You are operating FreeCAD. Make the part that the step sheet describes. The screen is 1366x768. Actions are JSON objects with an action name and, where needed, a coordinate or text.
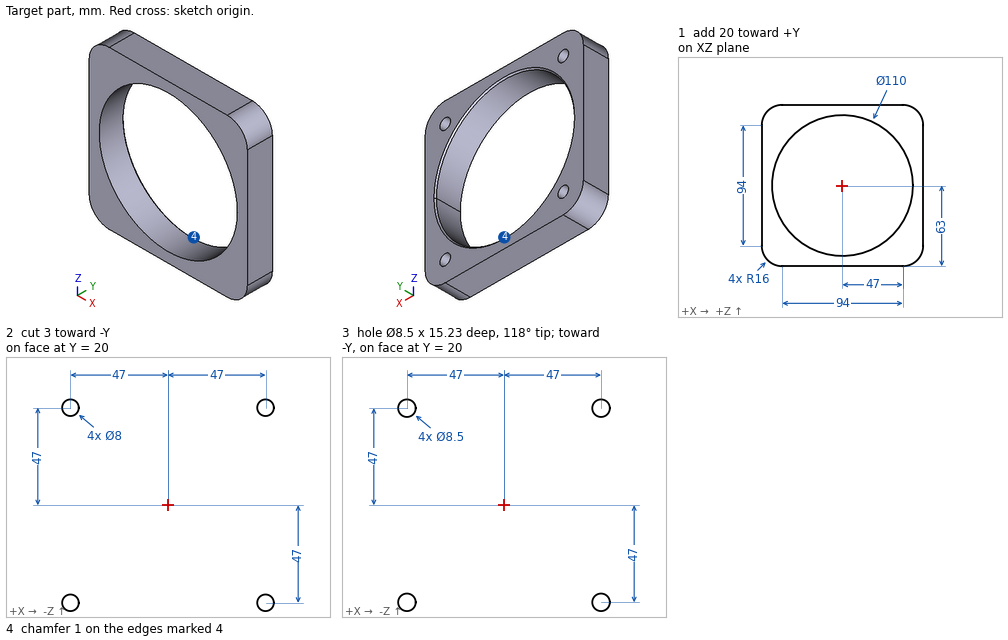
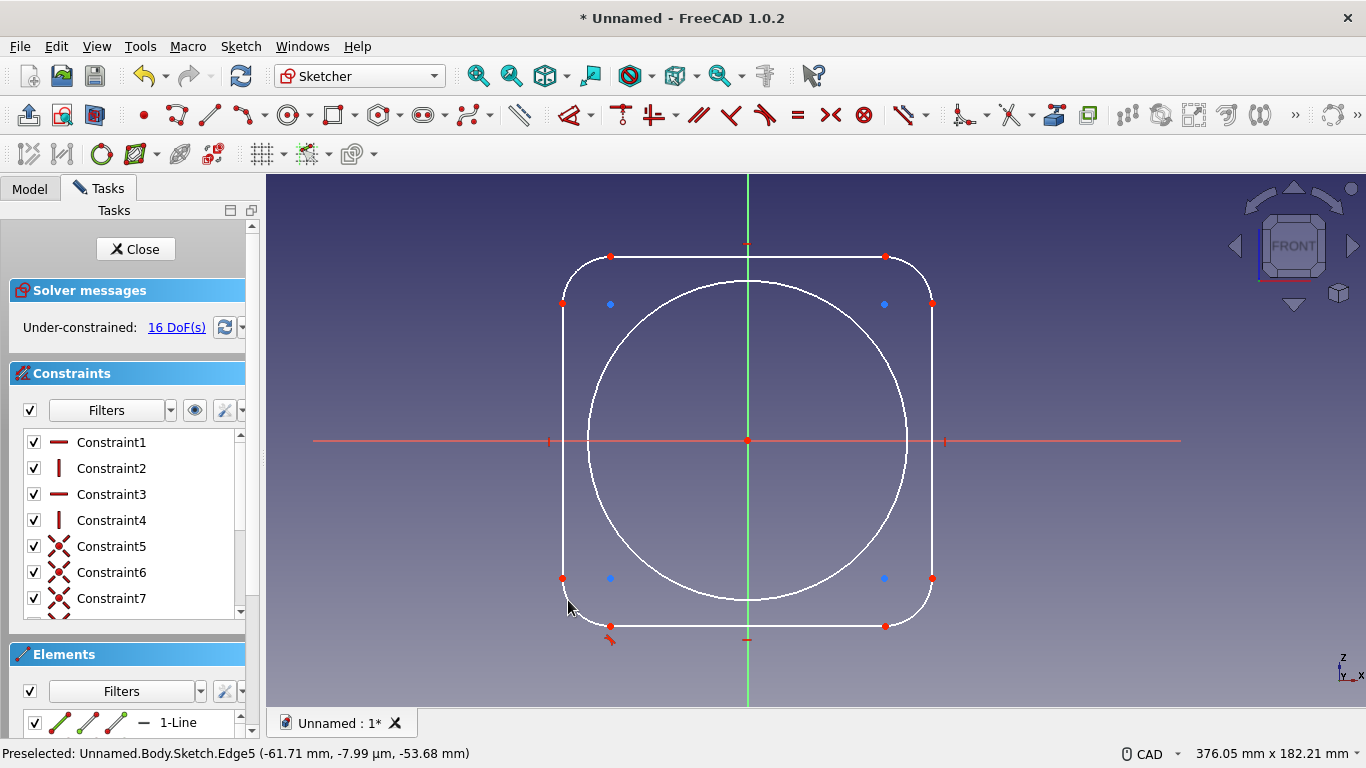
{"action": "left_click", "coordinate": [803, 626]}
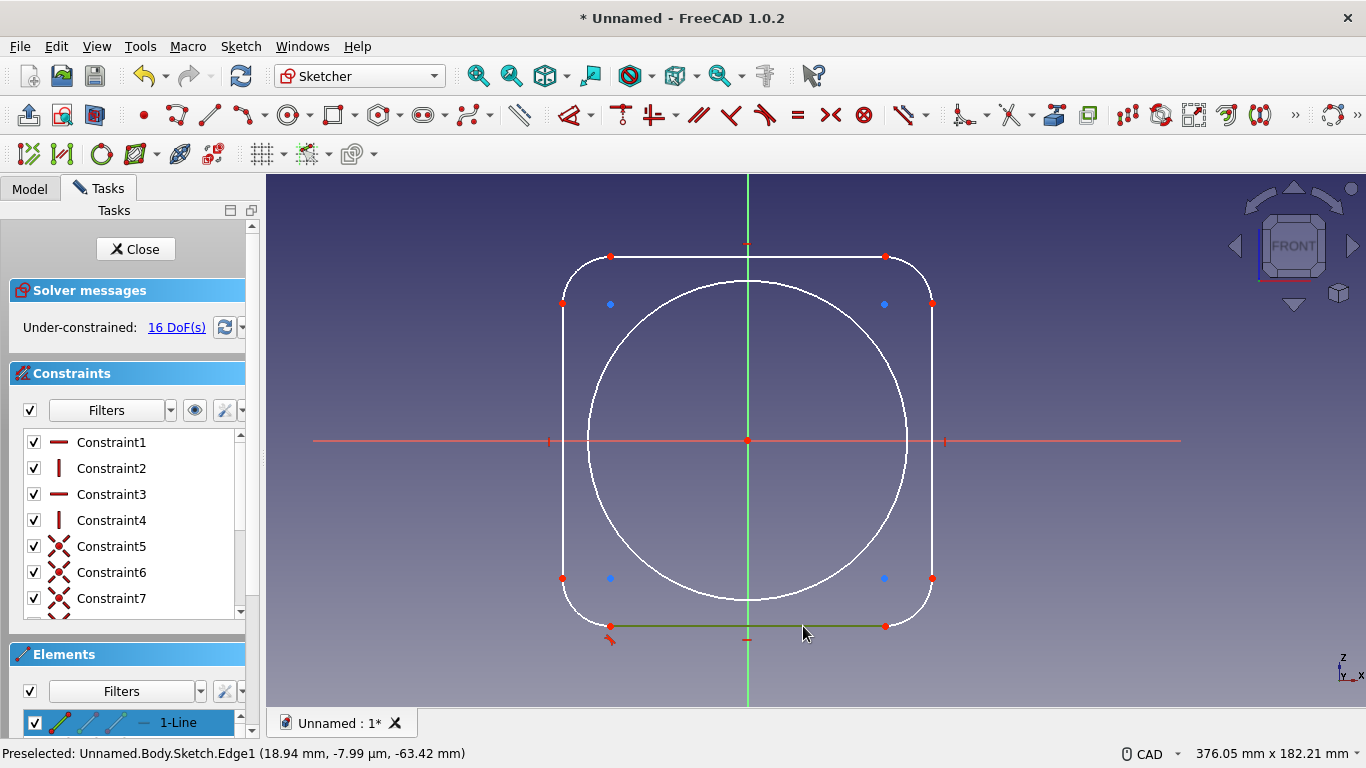
{"action": "left_click", "coordinate": [906, 621]}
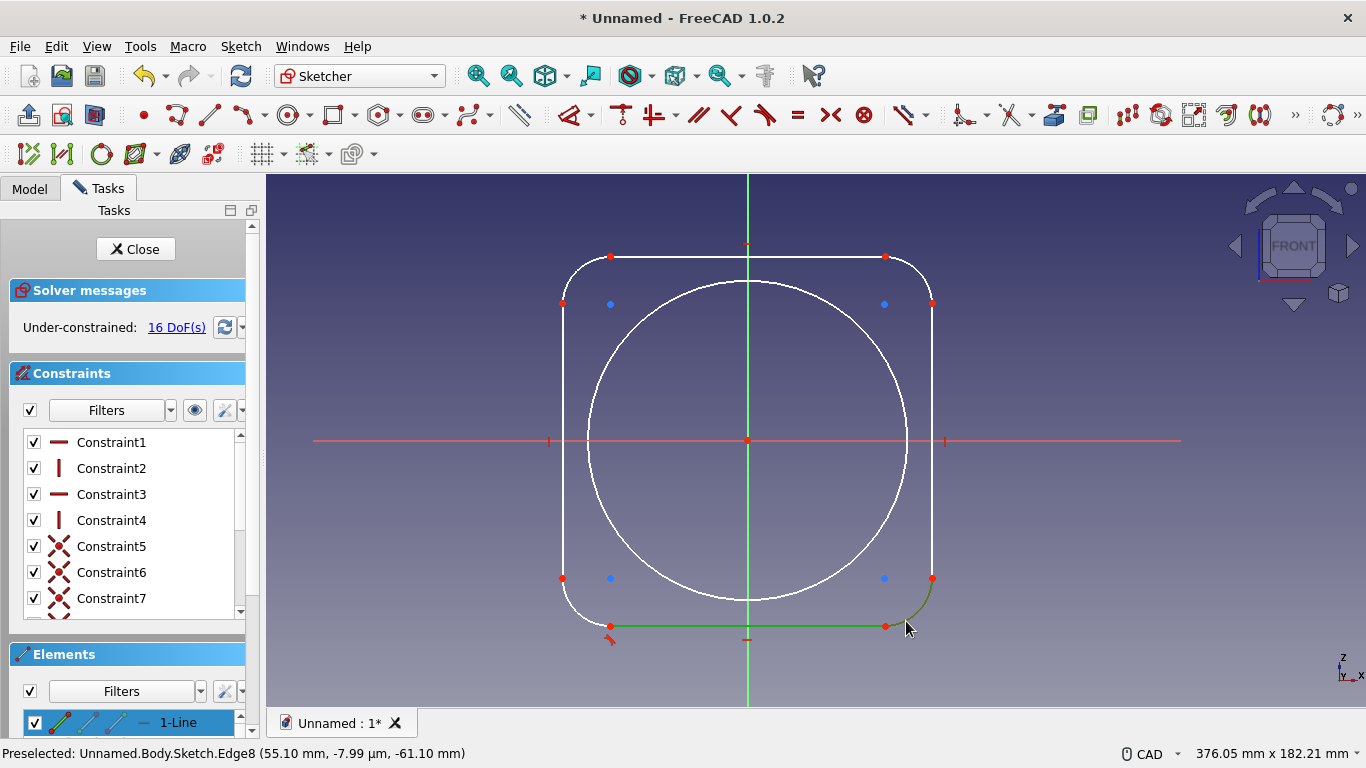
{"action": "left_click", "coordinate": [765, 116]}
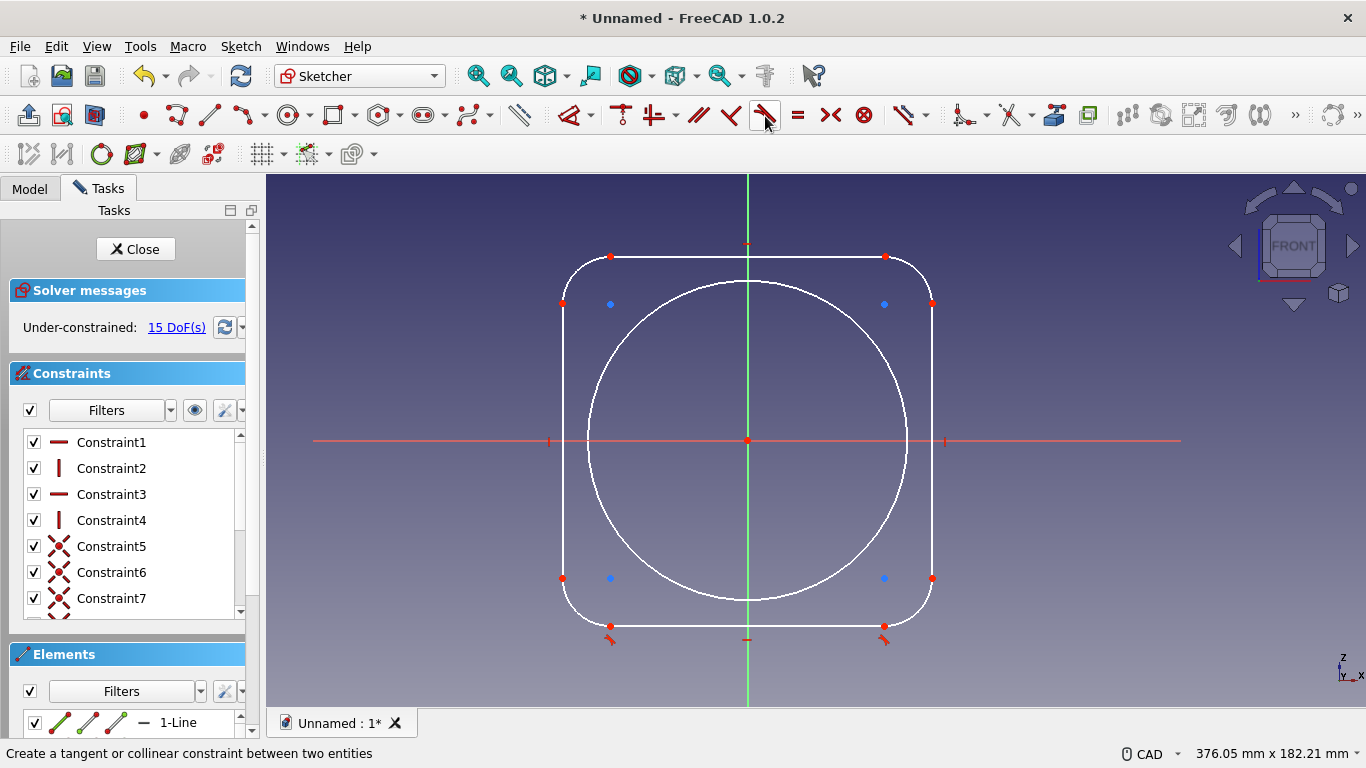
{"action": "left_click", "coordinate": [563, 496]}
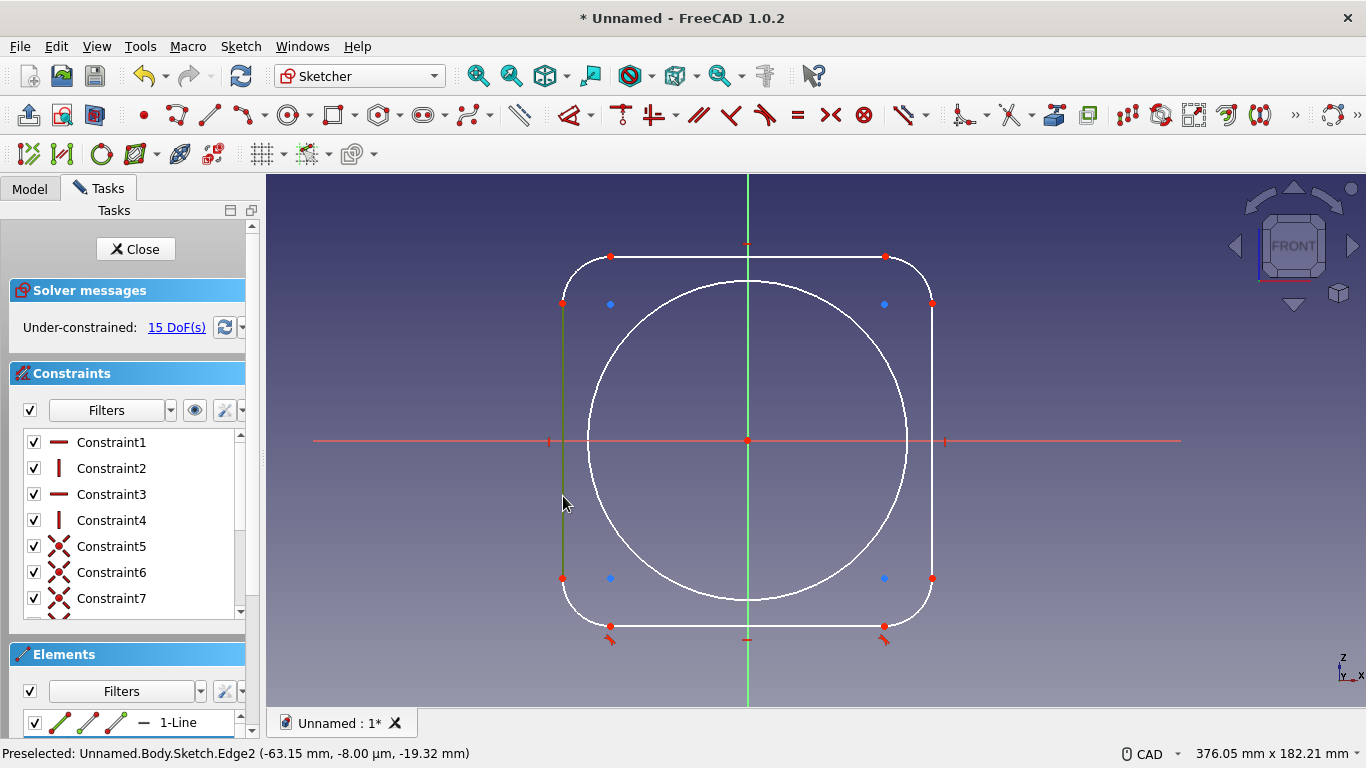
{"action": "left_click", "coordinate": [568, 600]}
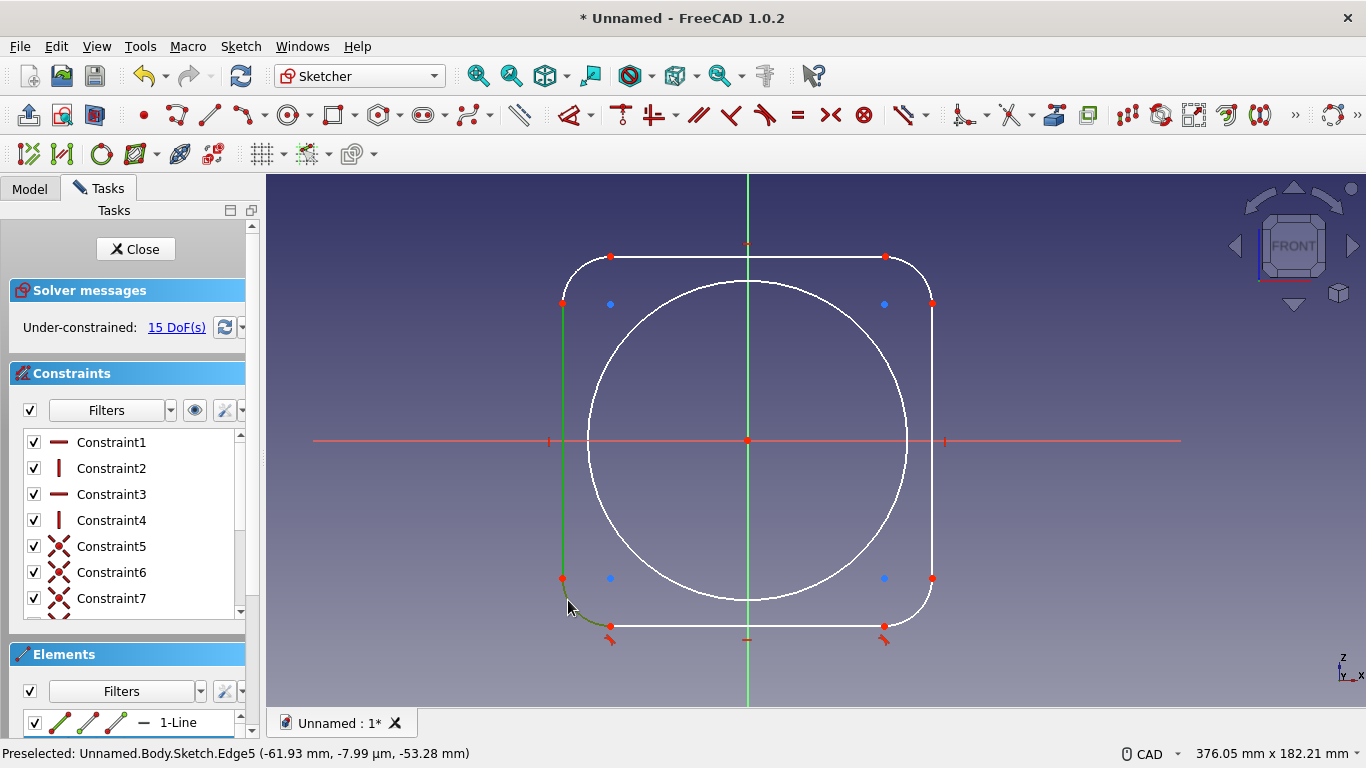
{"action": "key", "text": "t"}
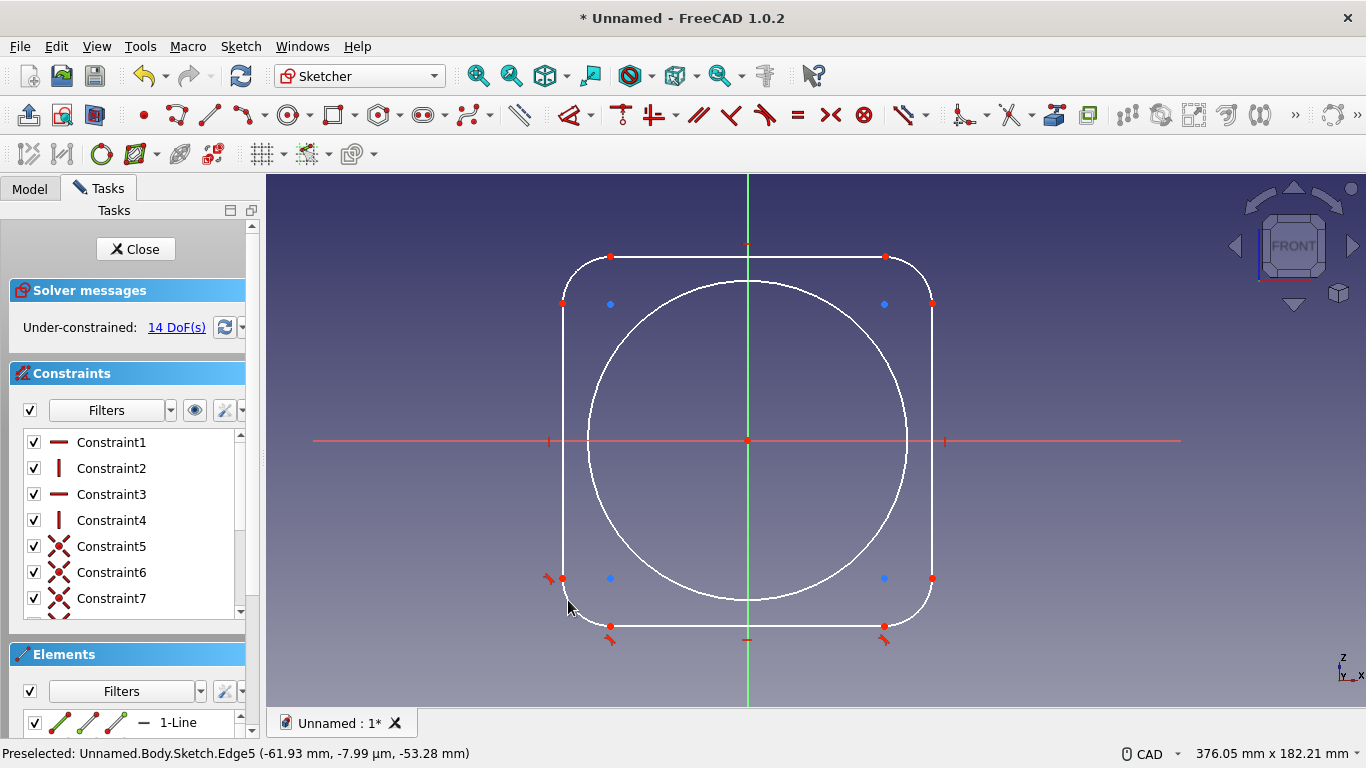
{"action": "left_click", "coordinate": [563, 496]}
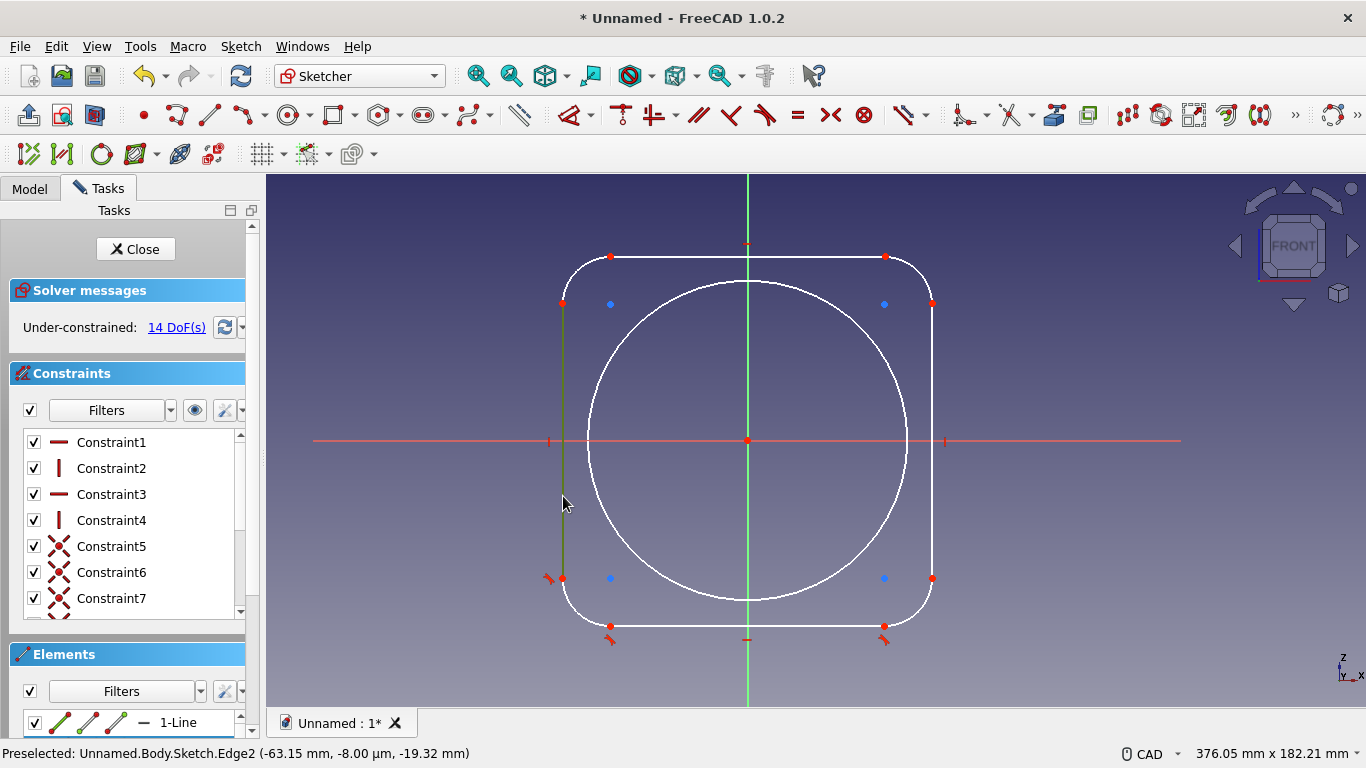
{"action": "left_click", "coordinate": [589, 262]}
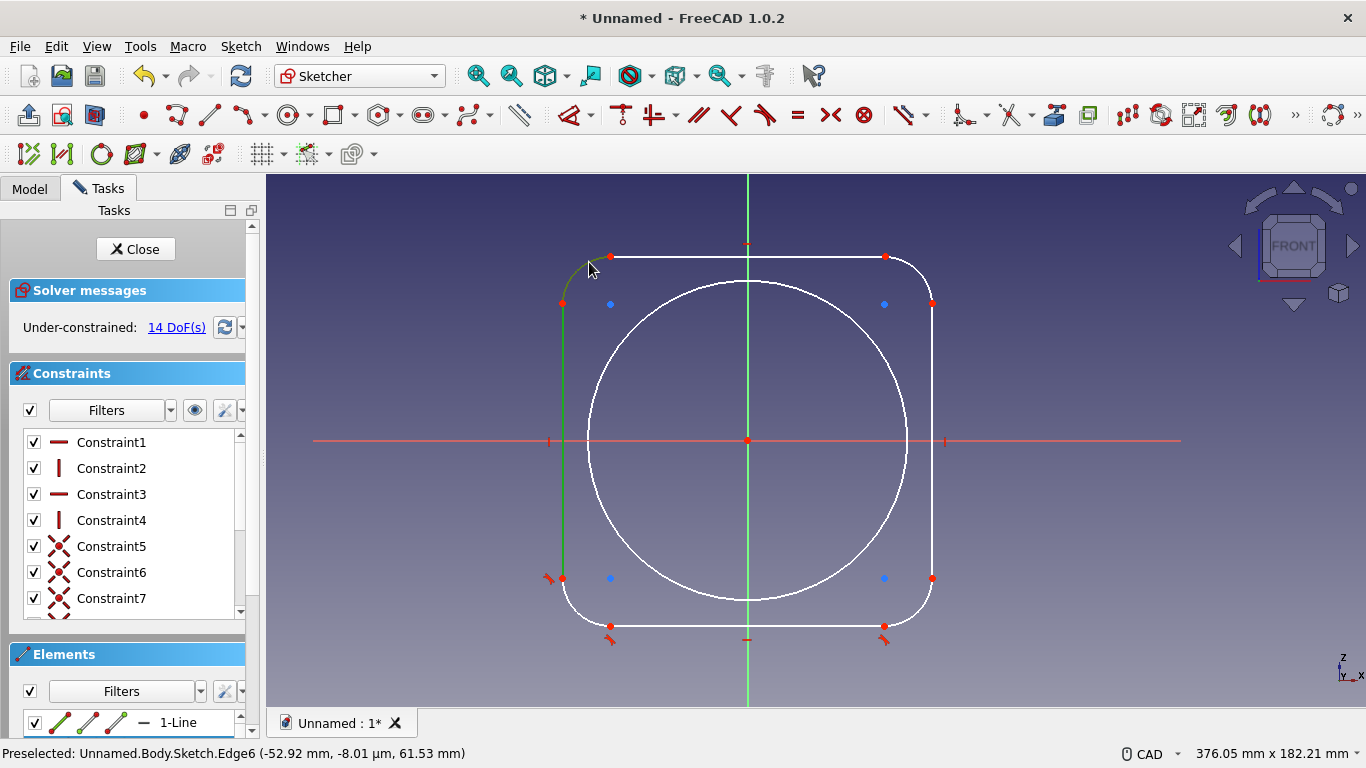
{"action": "left_click", "coordinate": [765, 116]}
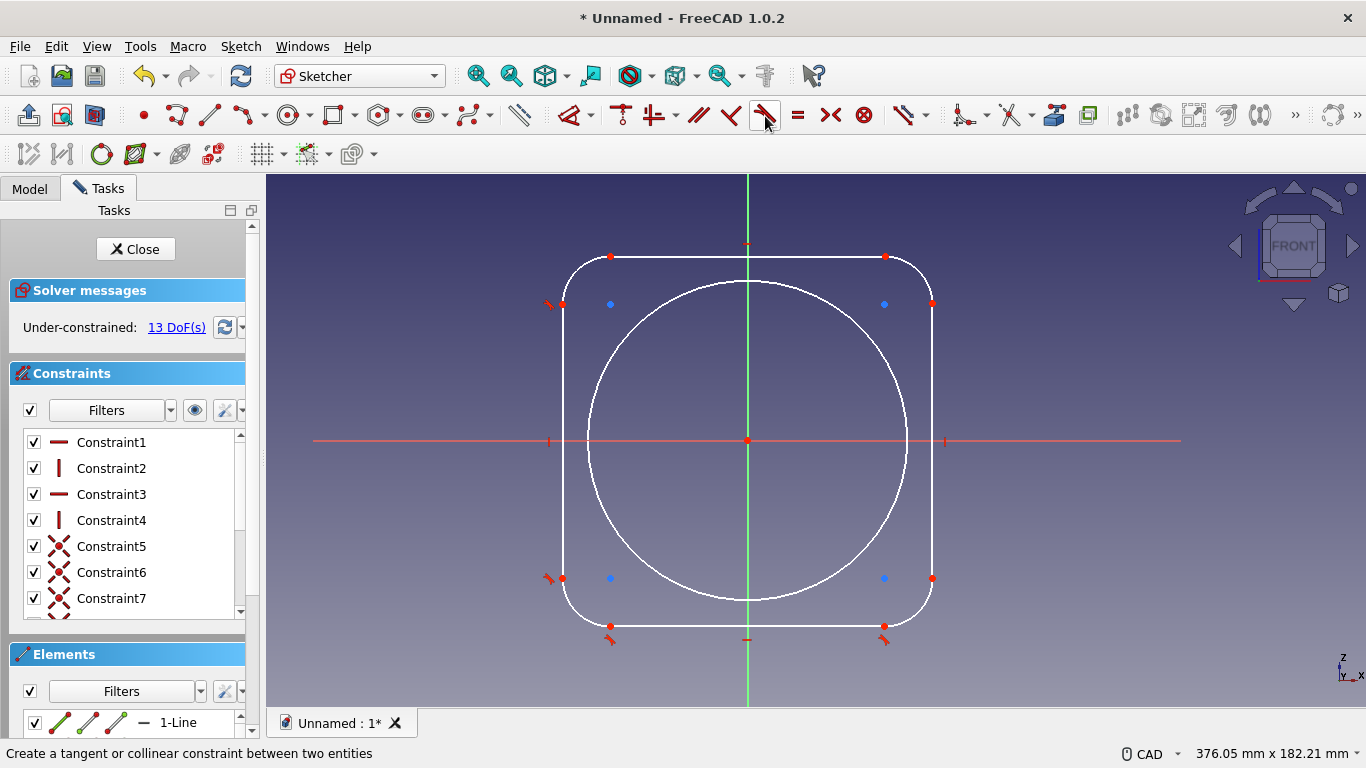
{"action": "left_click", "coordinate": [693, 257]}